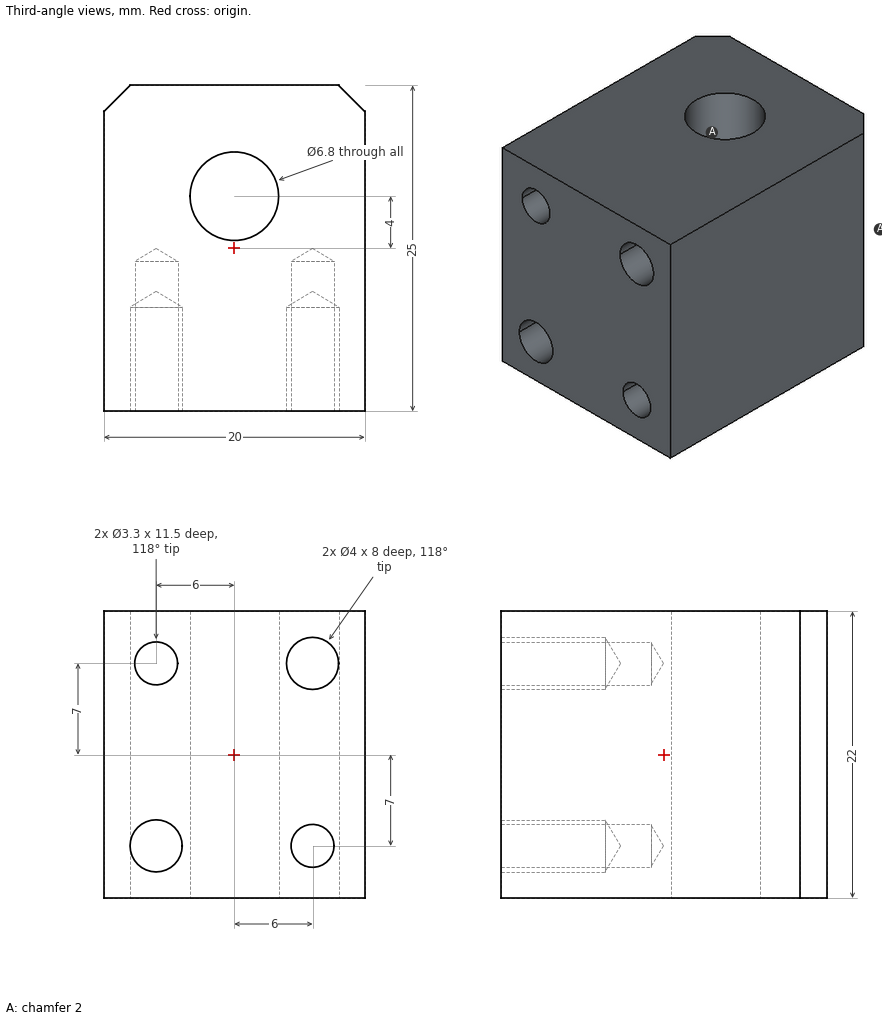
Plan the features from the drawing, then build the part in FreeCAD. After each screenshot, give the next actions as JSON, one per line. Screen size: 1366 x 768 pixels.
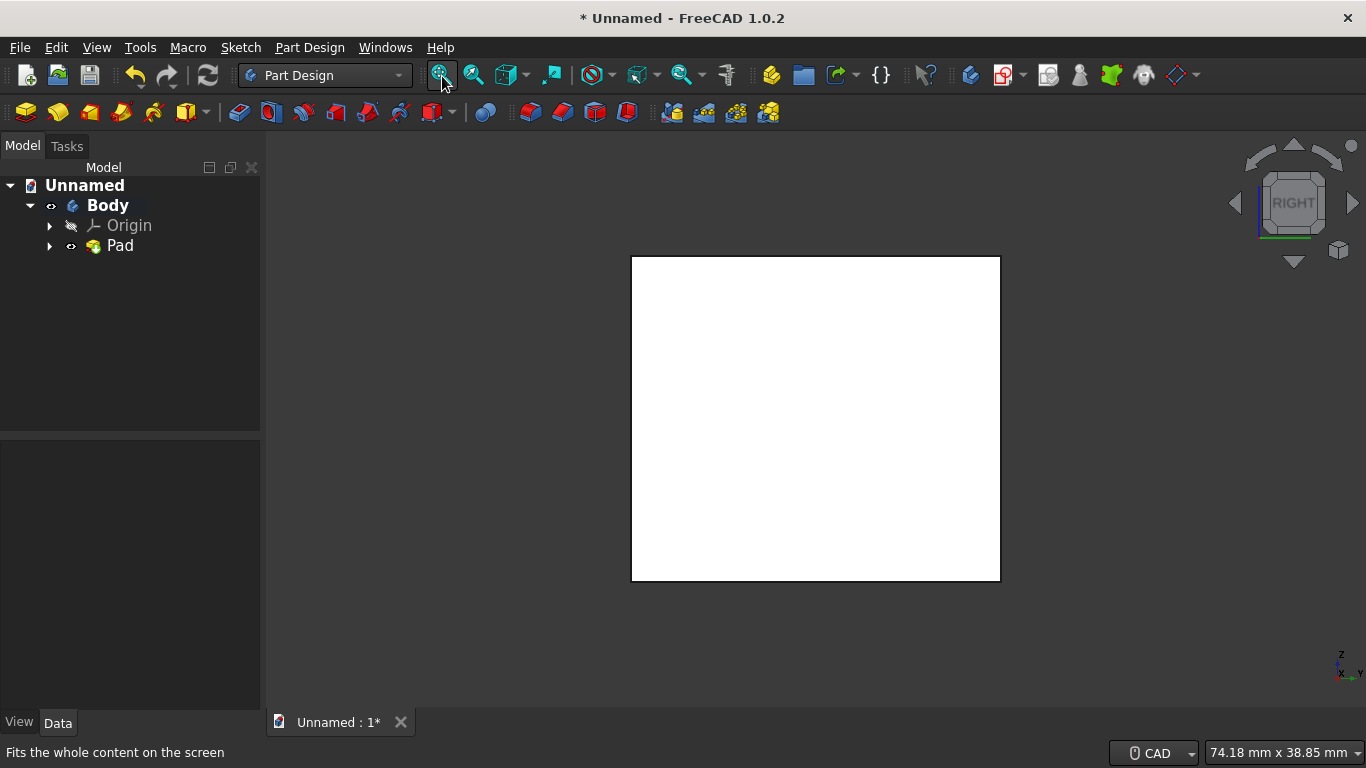
{"action": "left_click", "coordinate": [1001, 418]}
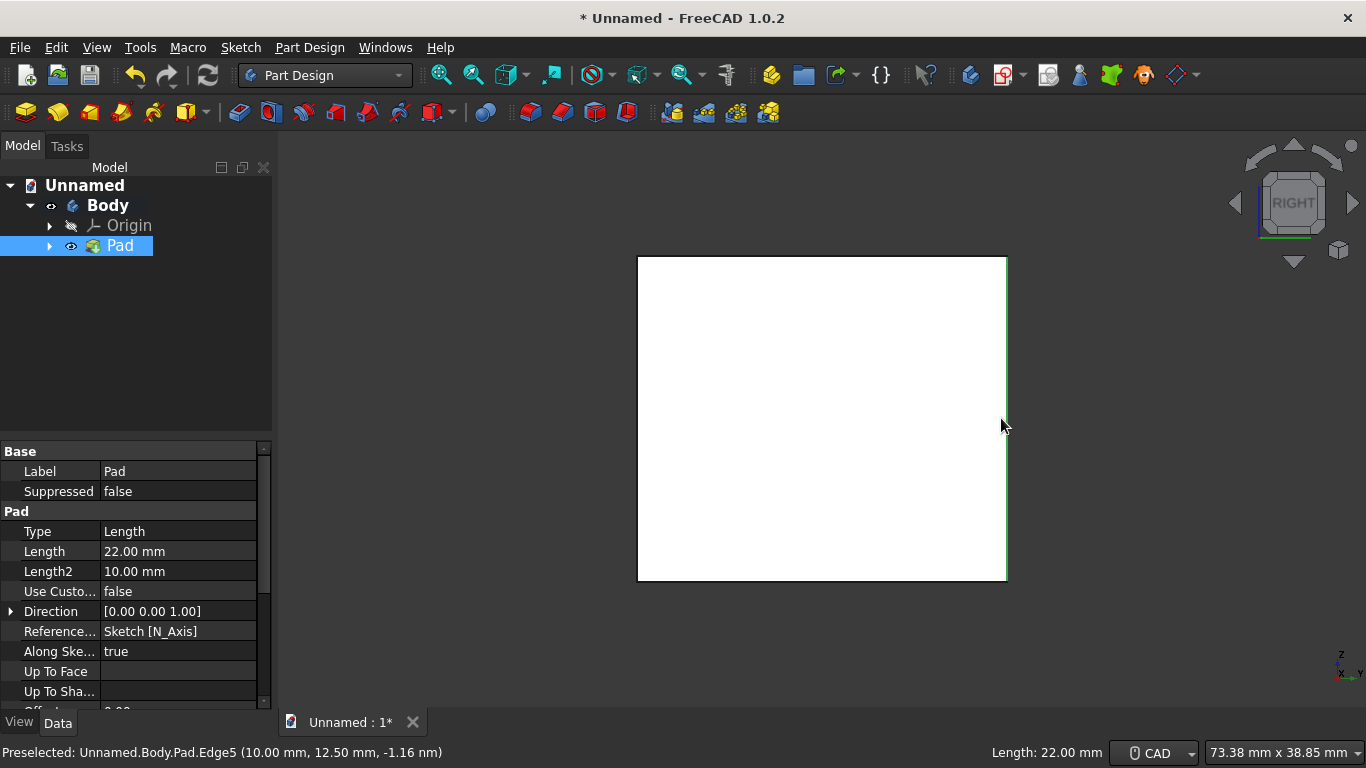
{"action": "key", "text": "5"}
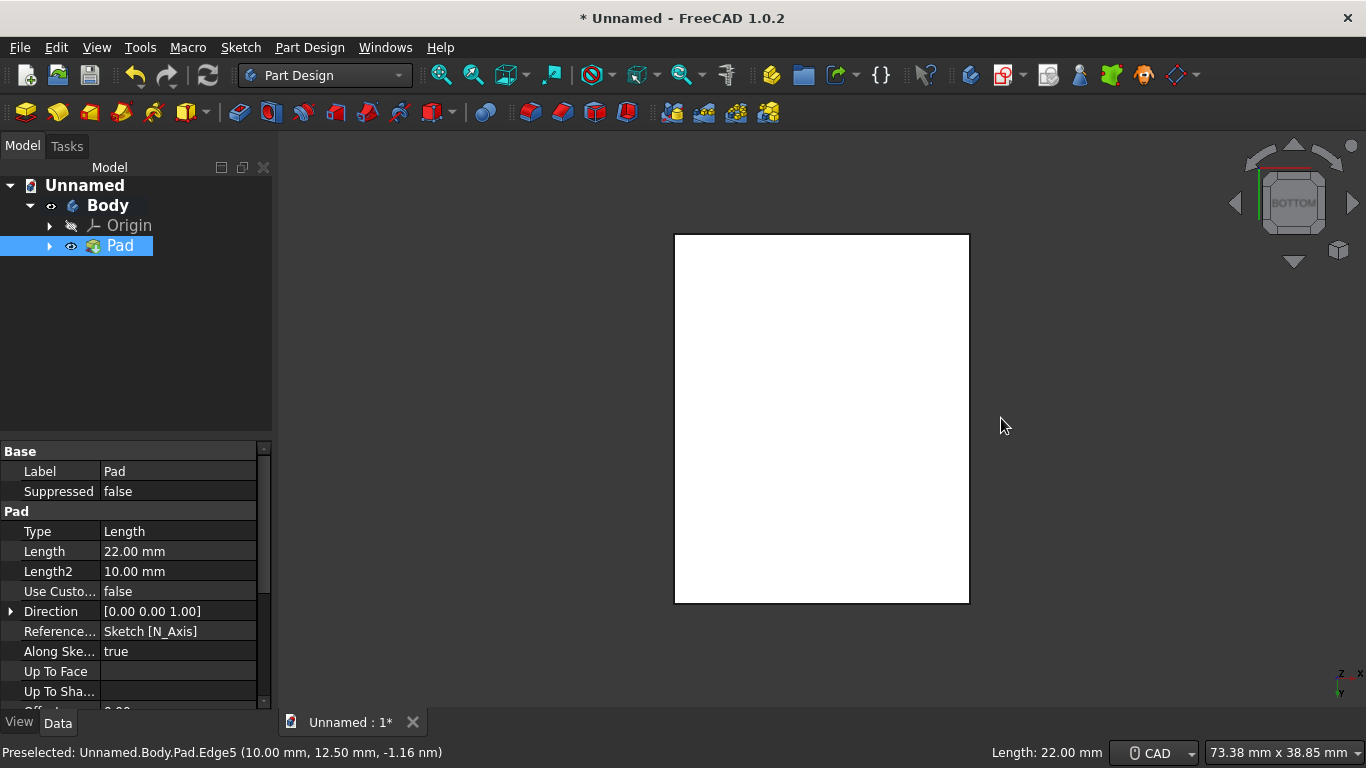
{"action": "key", "text": "4"}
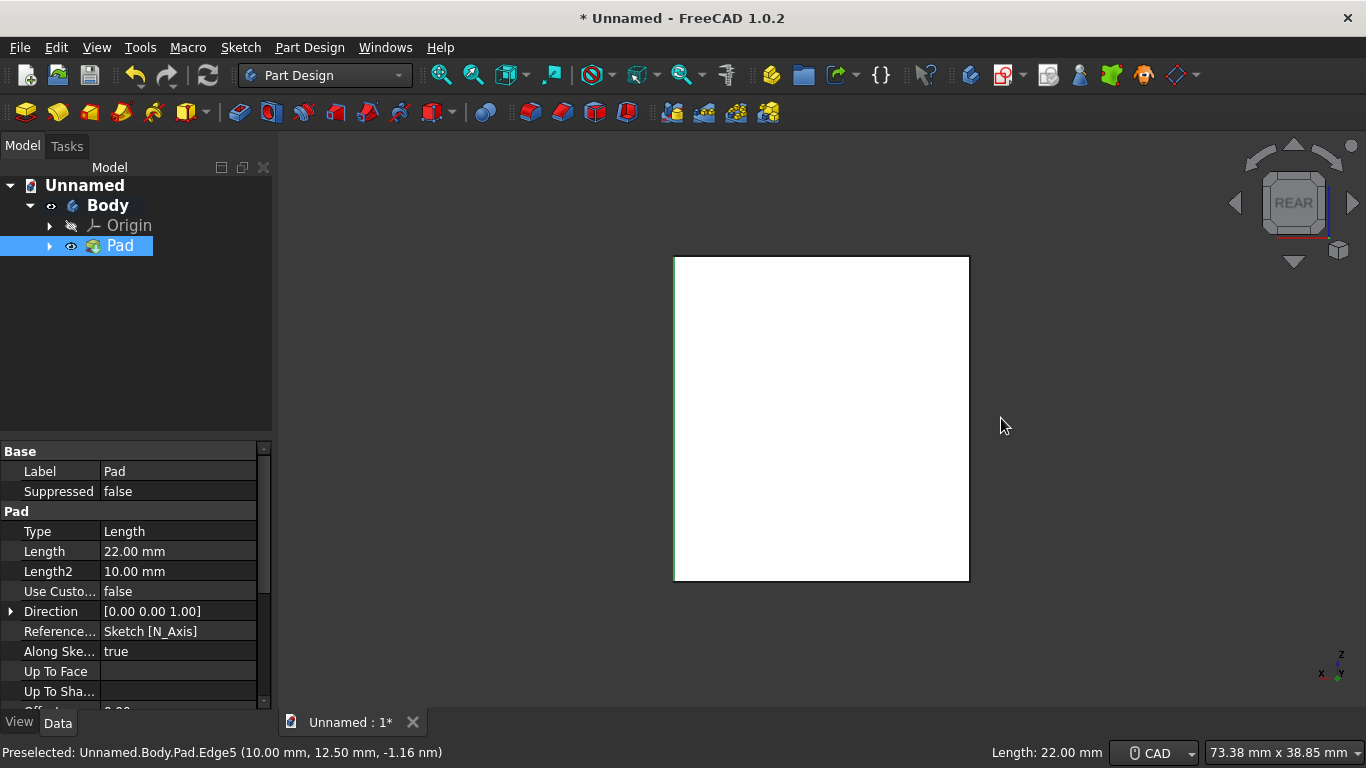
{"action": "left_click", "coordinate": [970, 418], "text": "ctrl"}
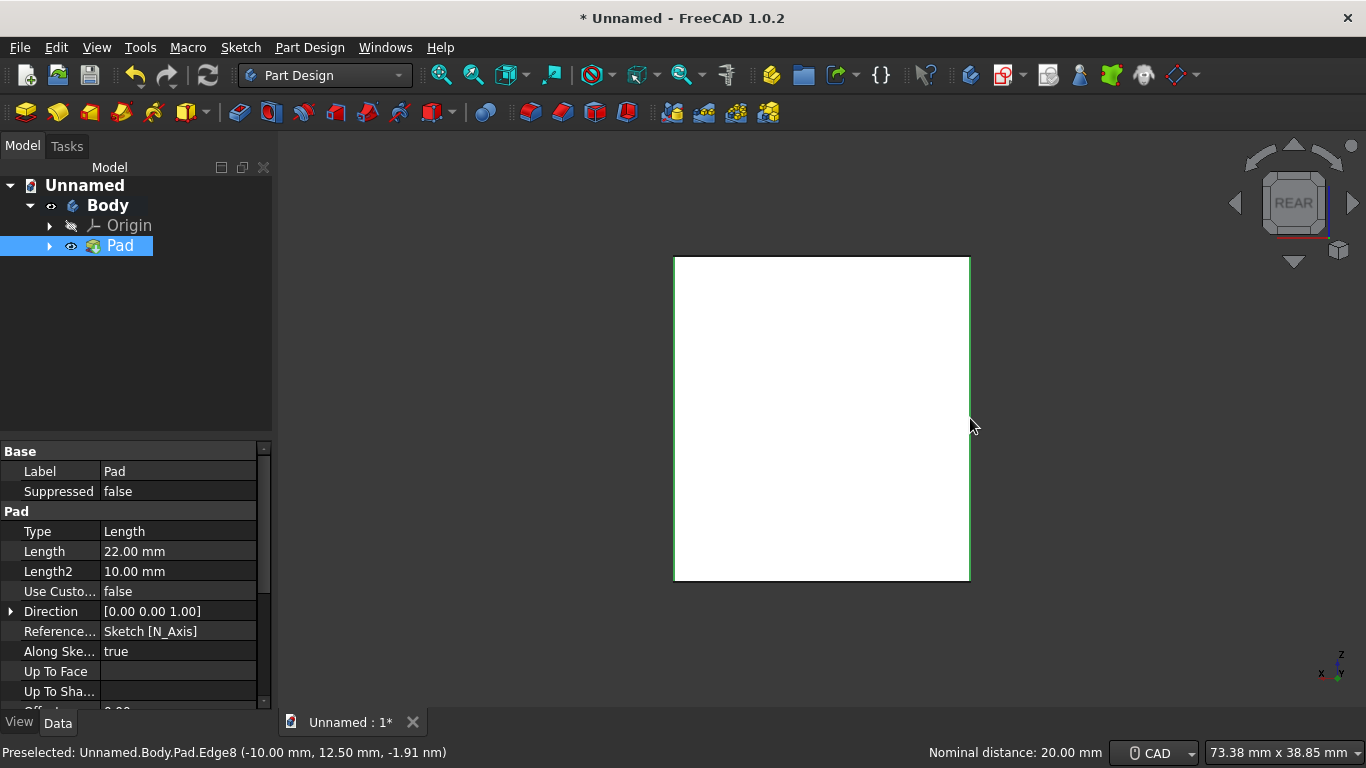
{"action": "left_click", "coordinate": [564, 112]}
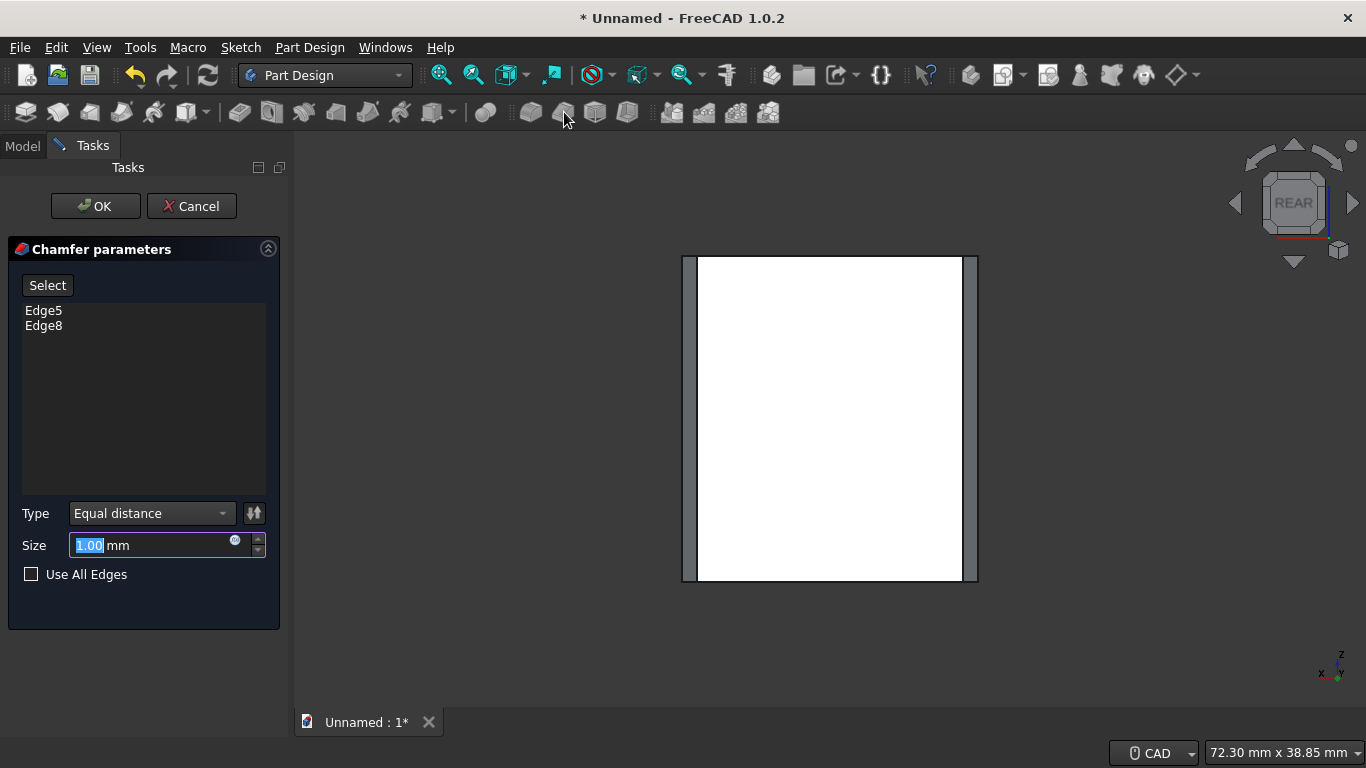
{"action": "type", "text": "2"}
{"action": "key", "text": "Tab"}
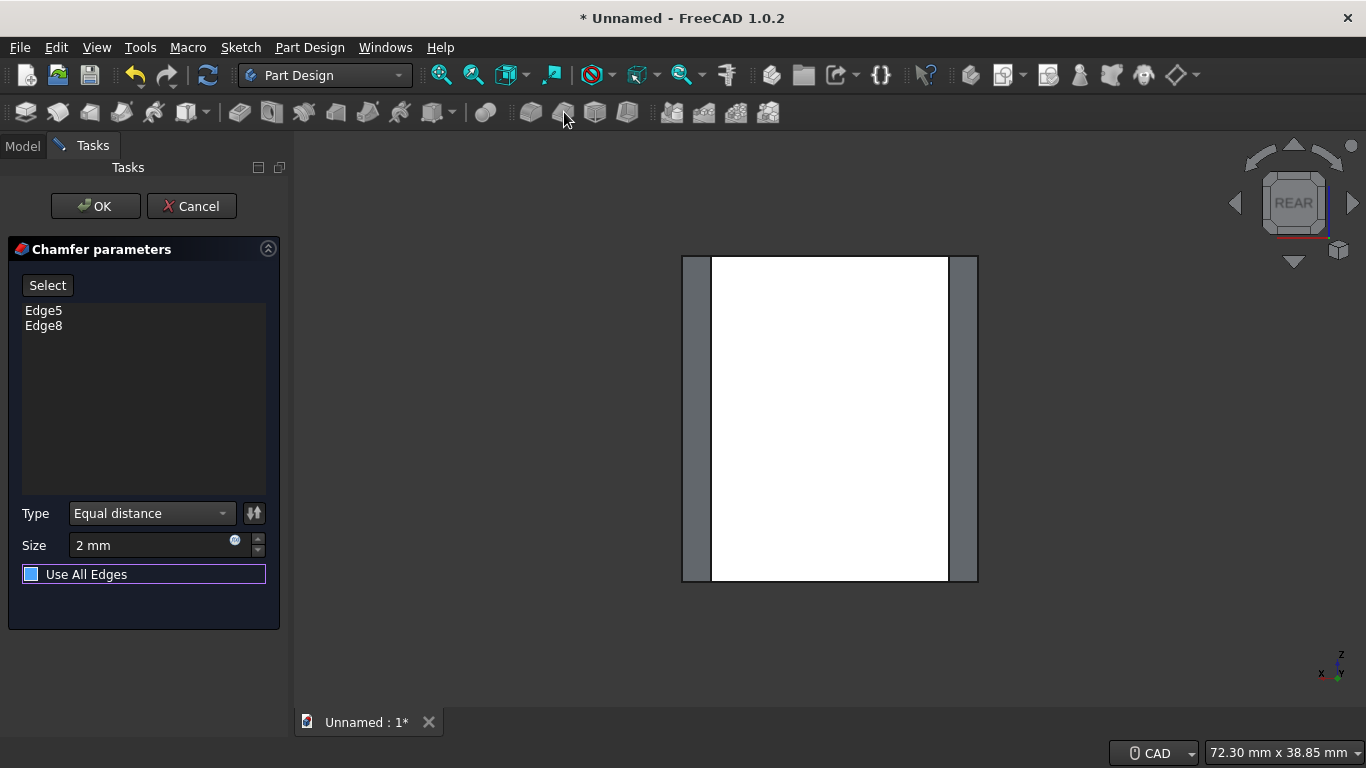
{"action": "left_click", "coordinate": [96, 206]}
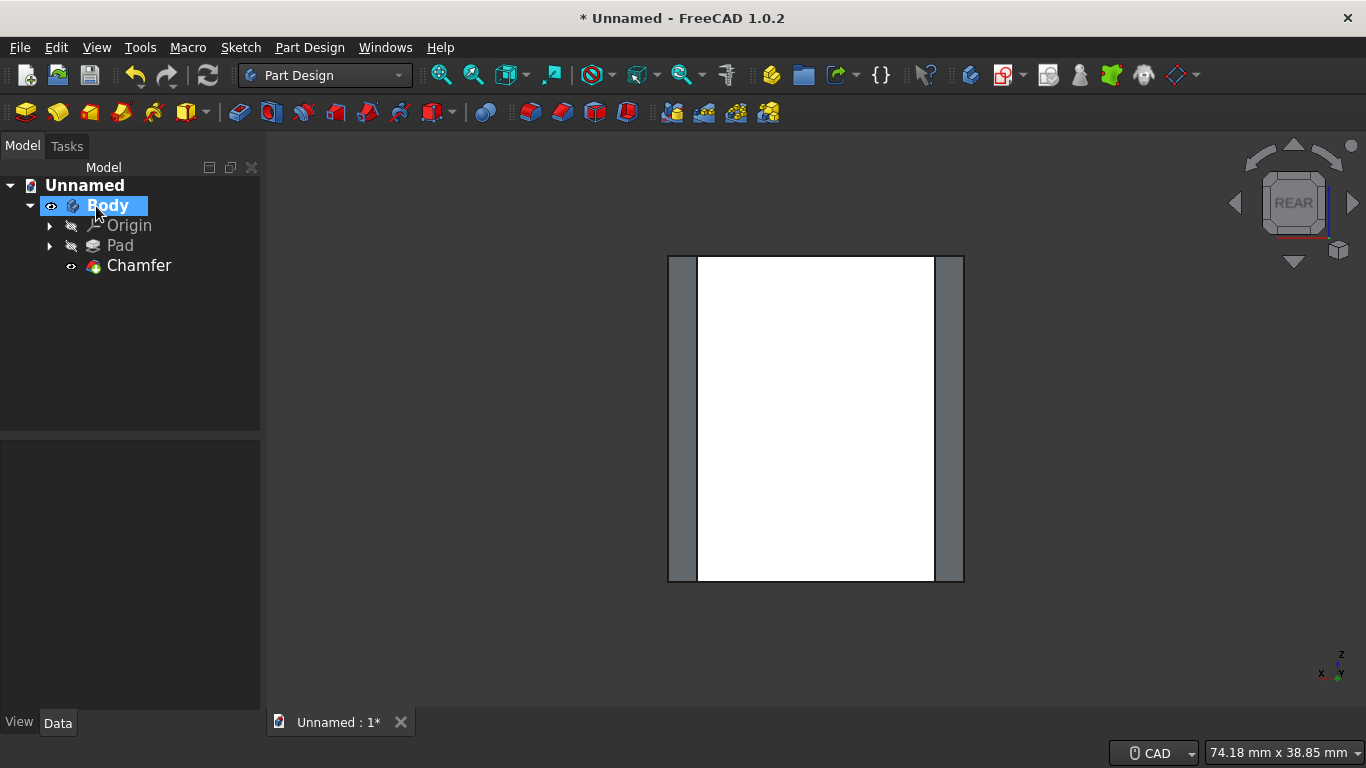
{"action": "key", "text": "0"}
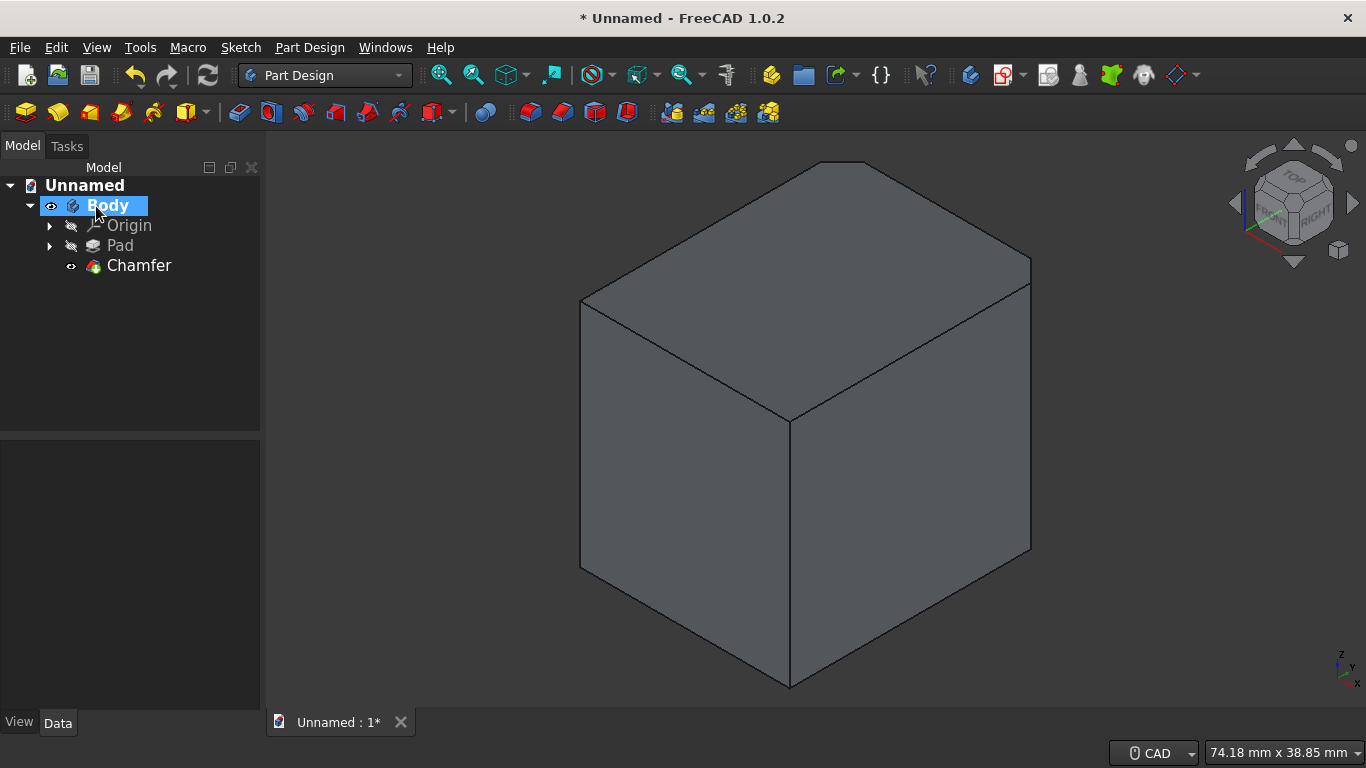
{"action": "left_click", "coordinate": [816, 285]}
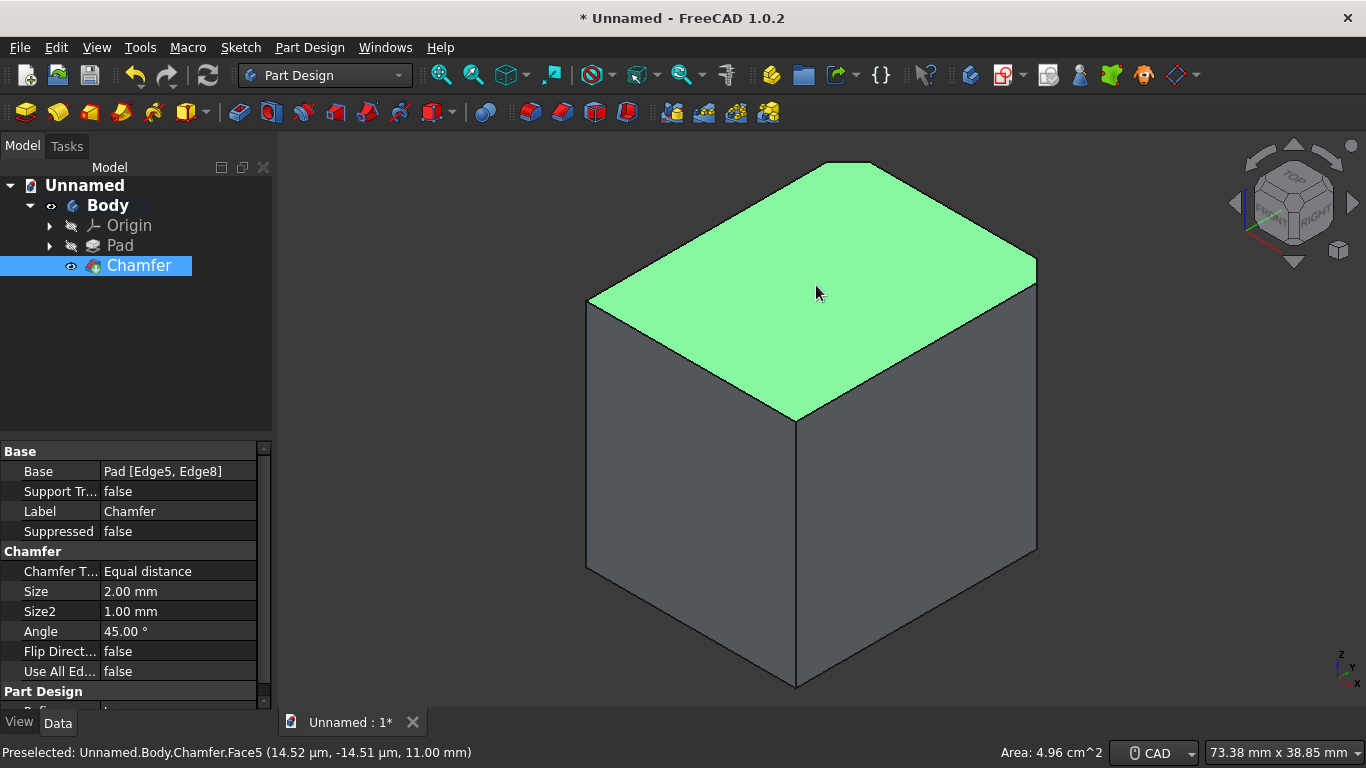
{"action": "left_click", "coordinate": [1004, 76]}